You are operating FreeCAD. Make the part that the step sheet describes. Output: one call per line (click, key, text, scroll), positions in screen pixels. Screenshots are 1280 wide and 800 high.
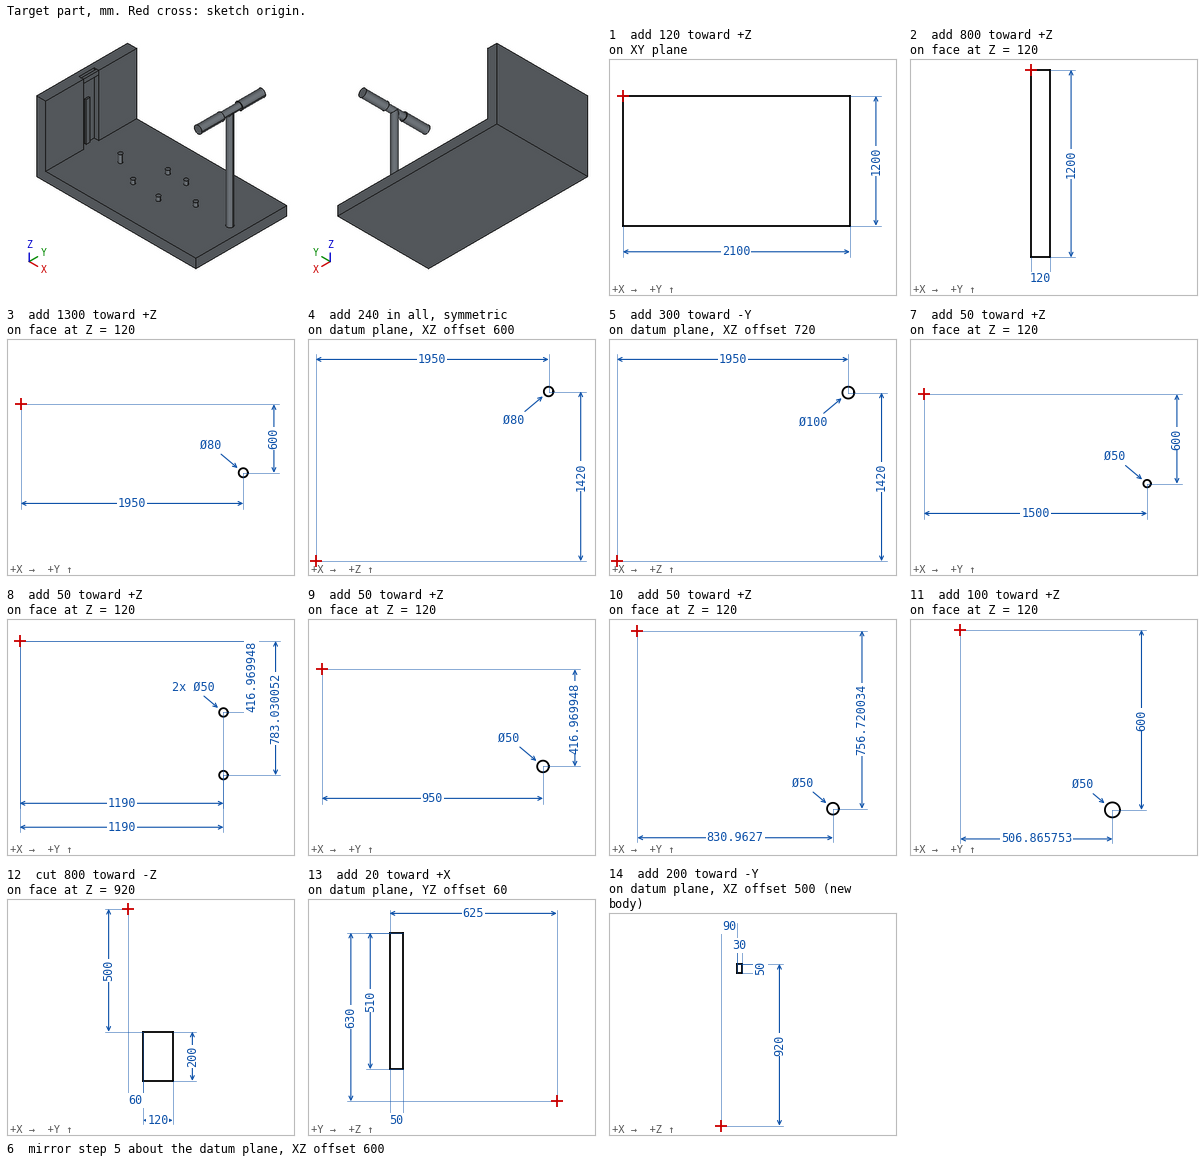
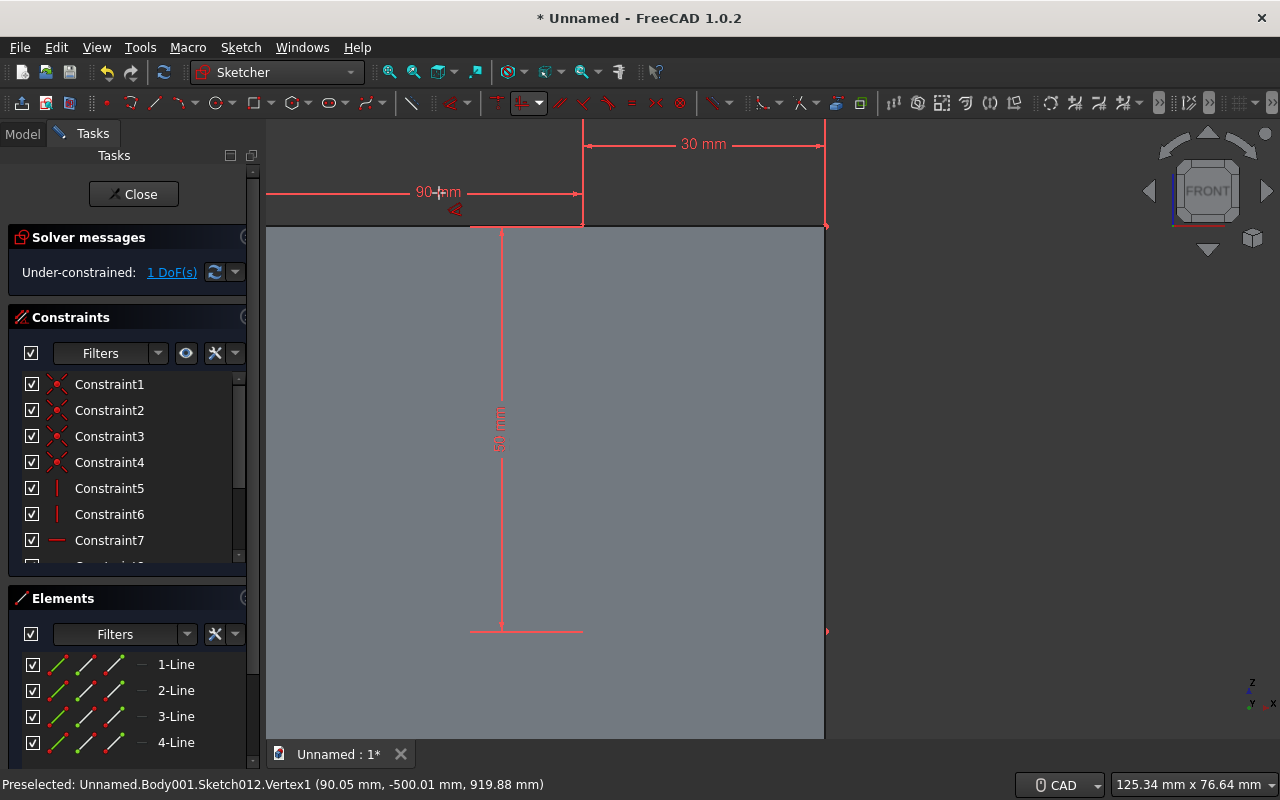
click(583, 227)
click(617, 469)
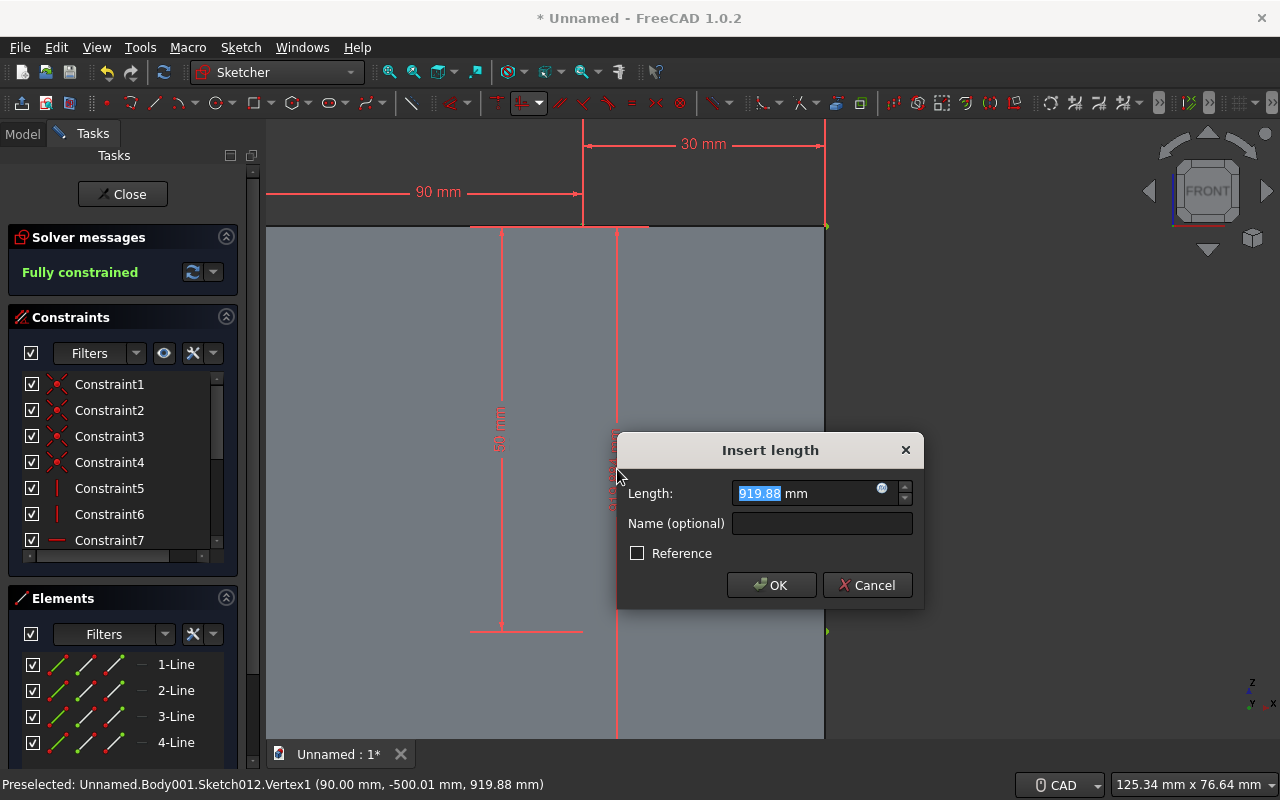
text(920)
key(Return)
key(Escape)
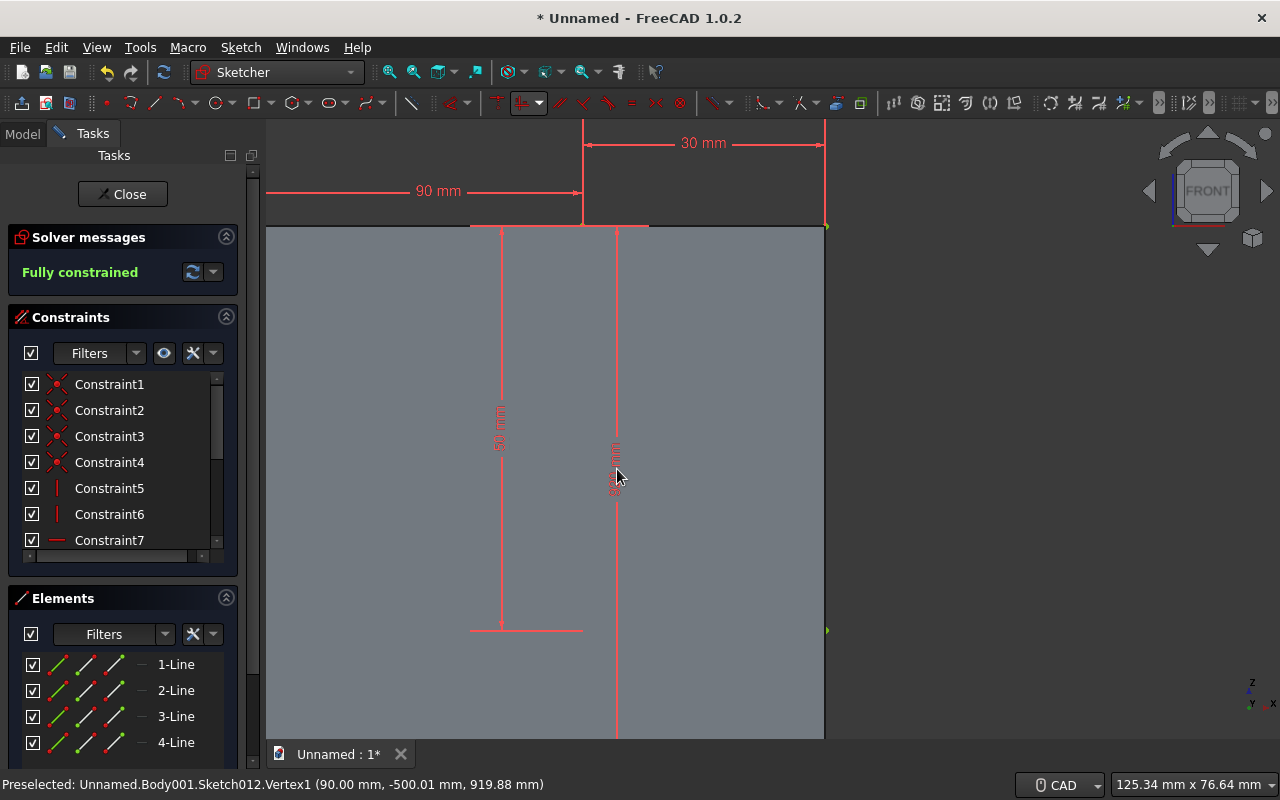
click(123, 194)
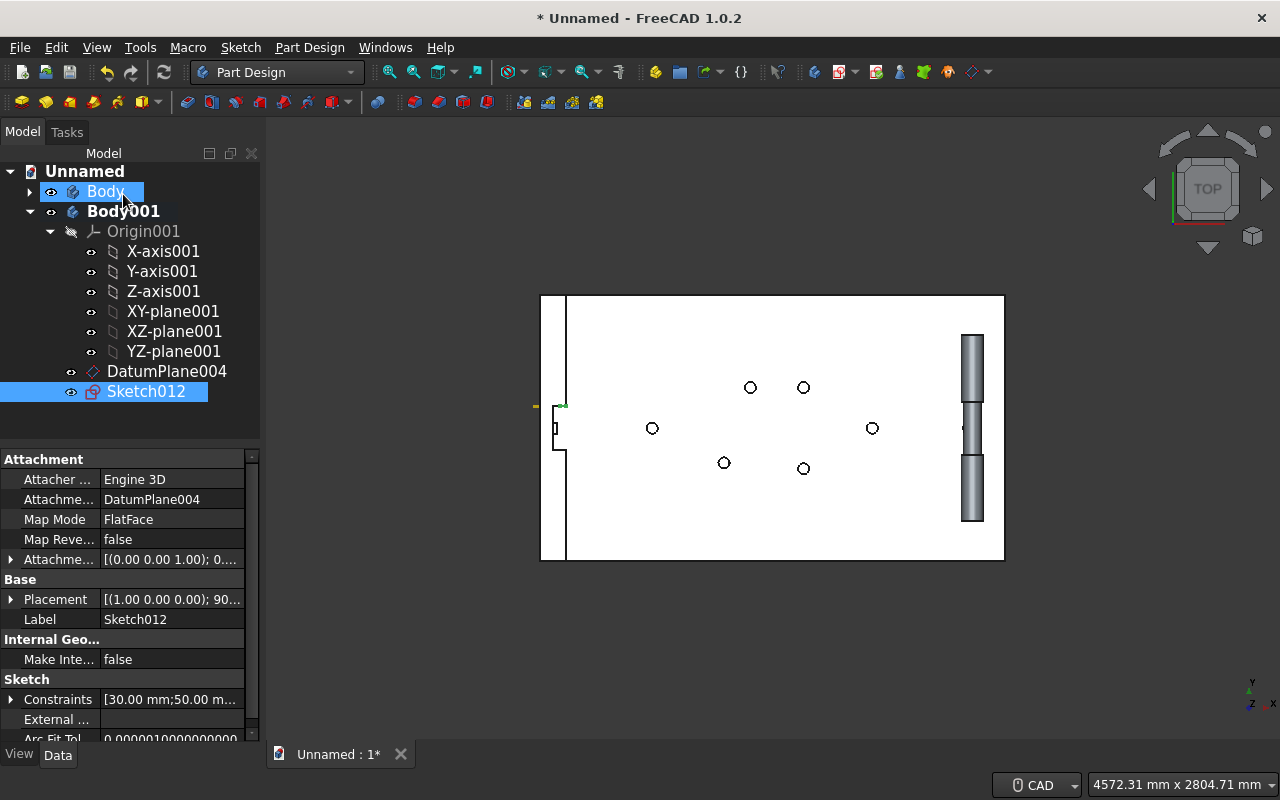
click(22, 102)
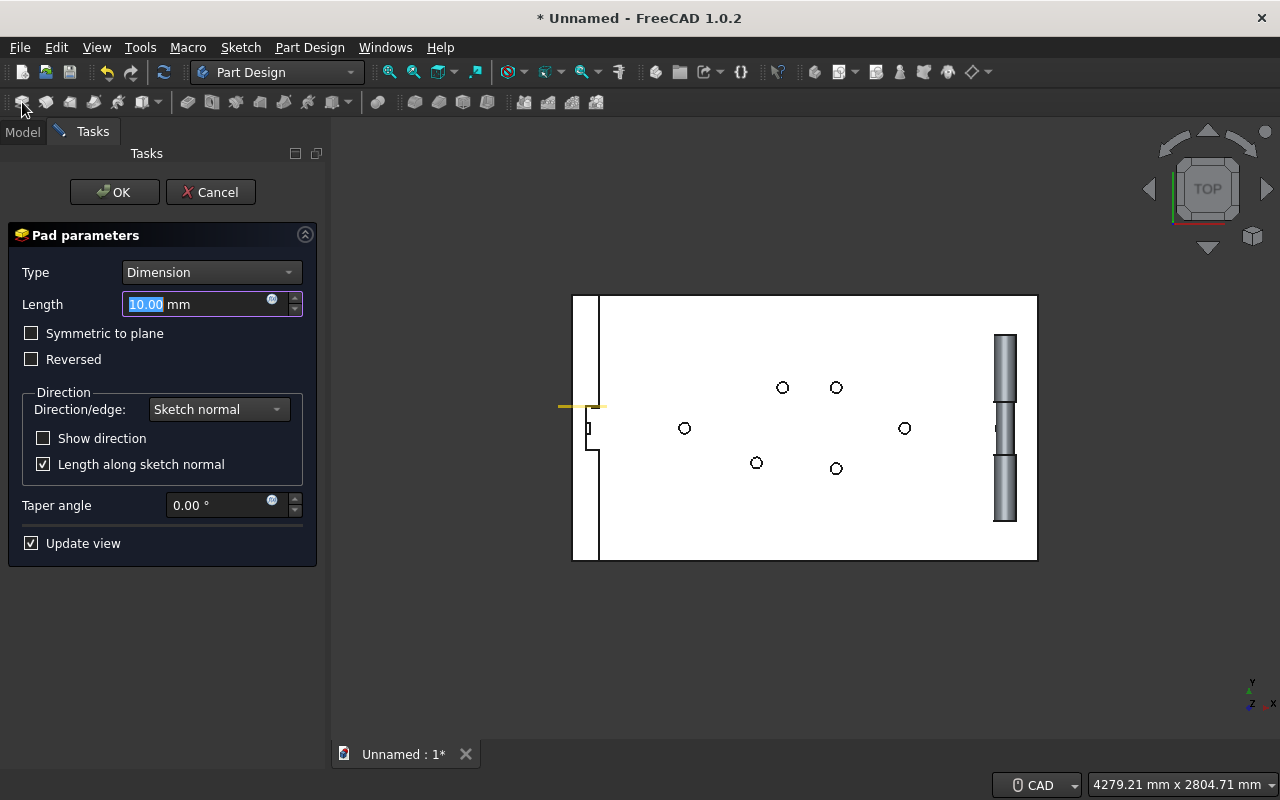
text(200)
key(Tab)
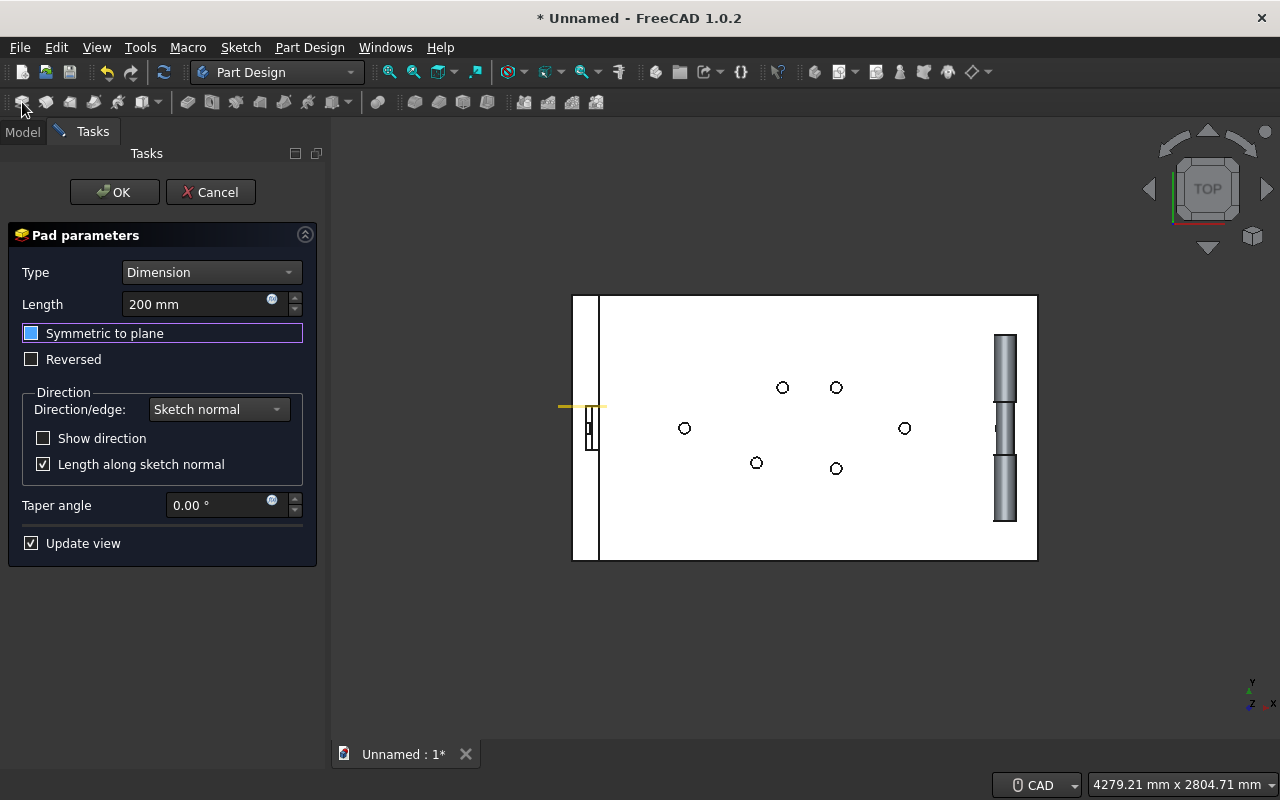
click(115, 192)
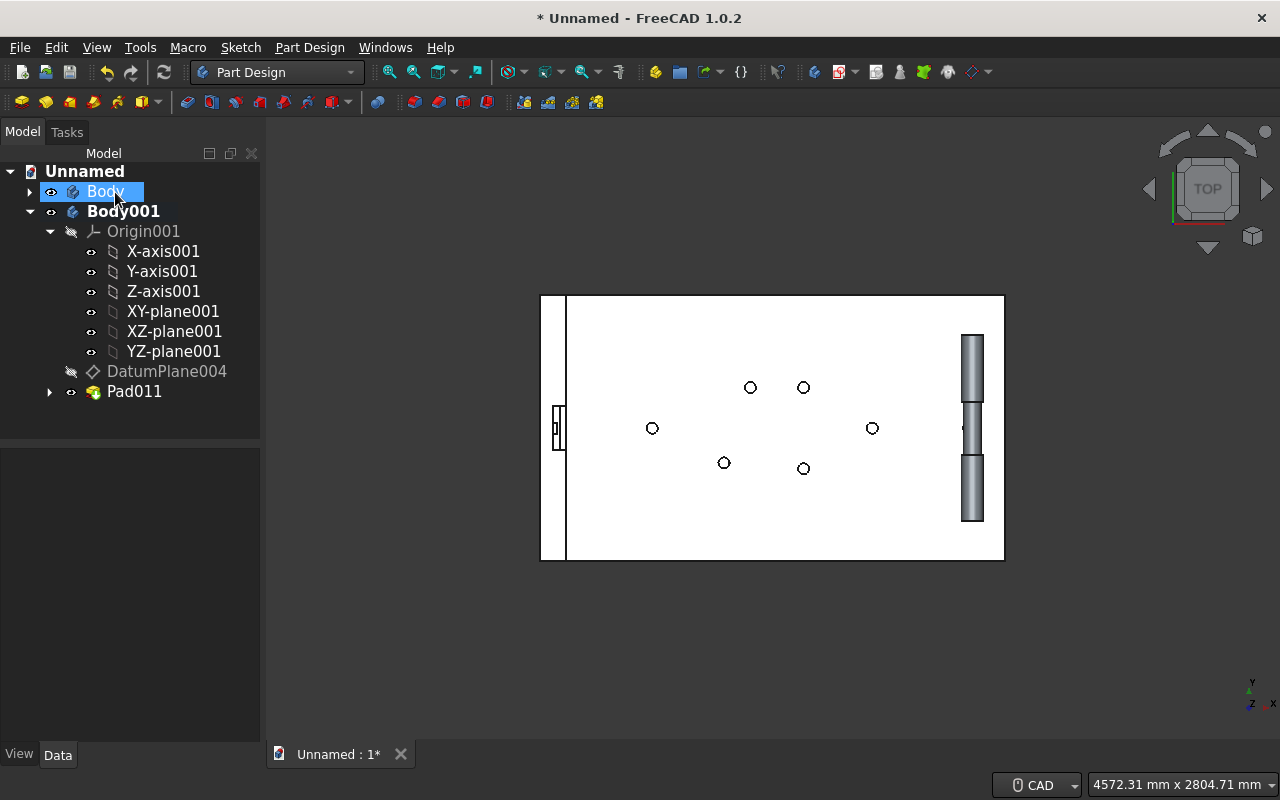
key(0)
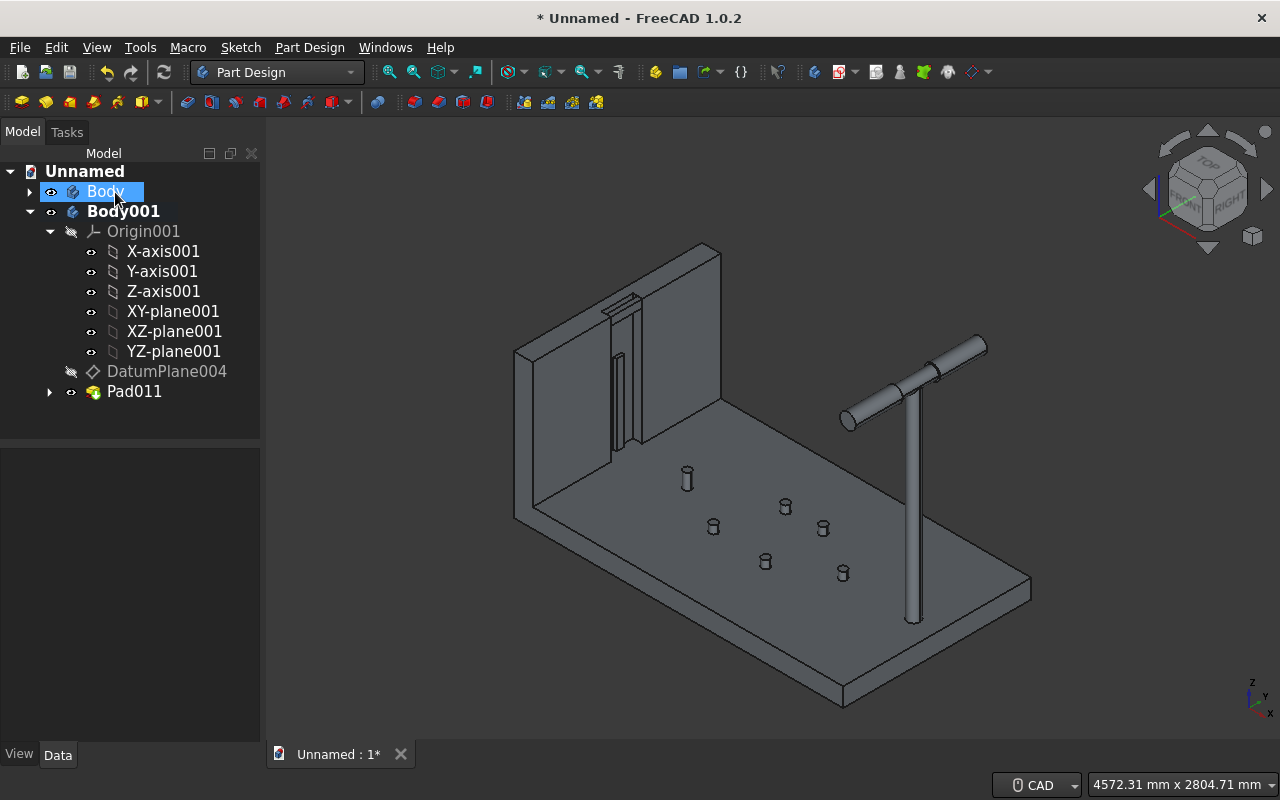
click(390, 72)